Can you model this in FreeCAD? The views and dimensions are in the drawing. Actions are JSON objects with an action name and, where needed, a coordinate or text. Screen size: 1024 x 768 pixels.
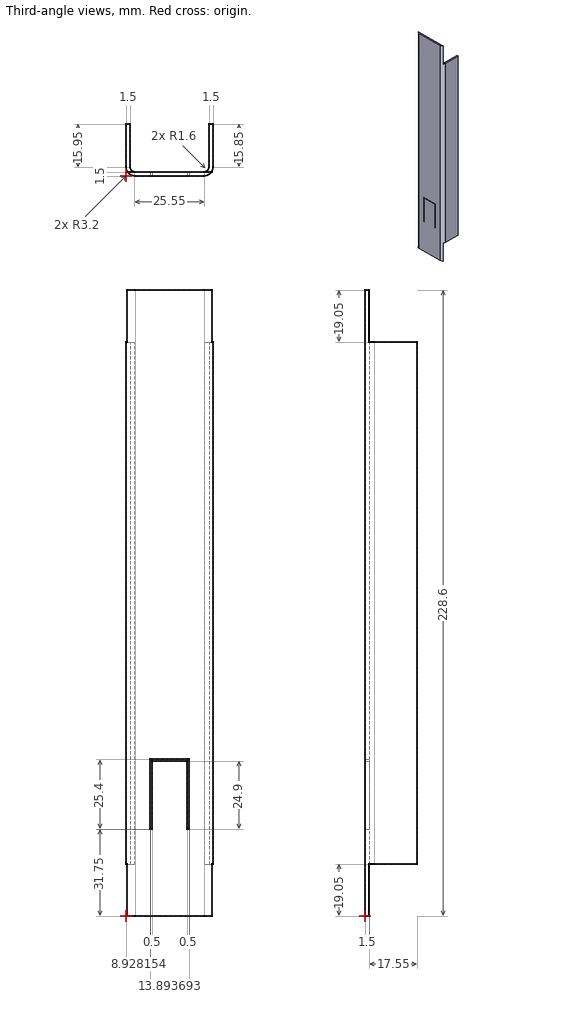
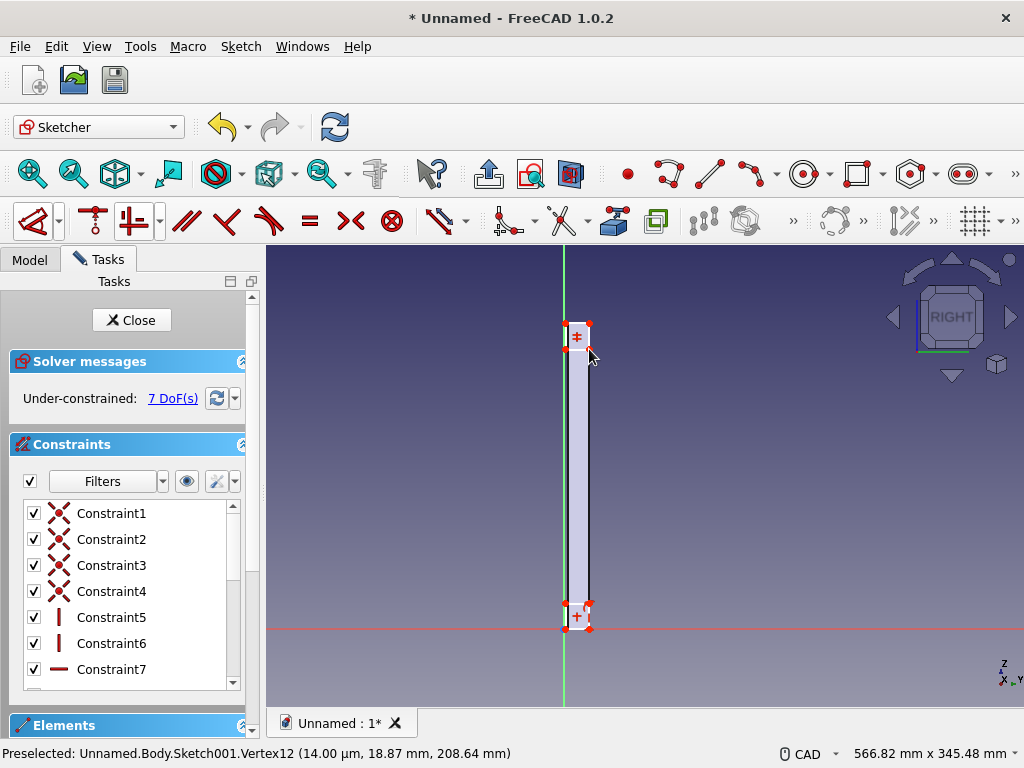
{"action": "scroll", "coordinate": [566, 604], "scroll_direction": "up", "scroll_amount": 15}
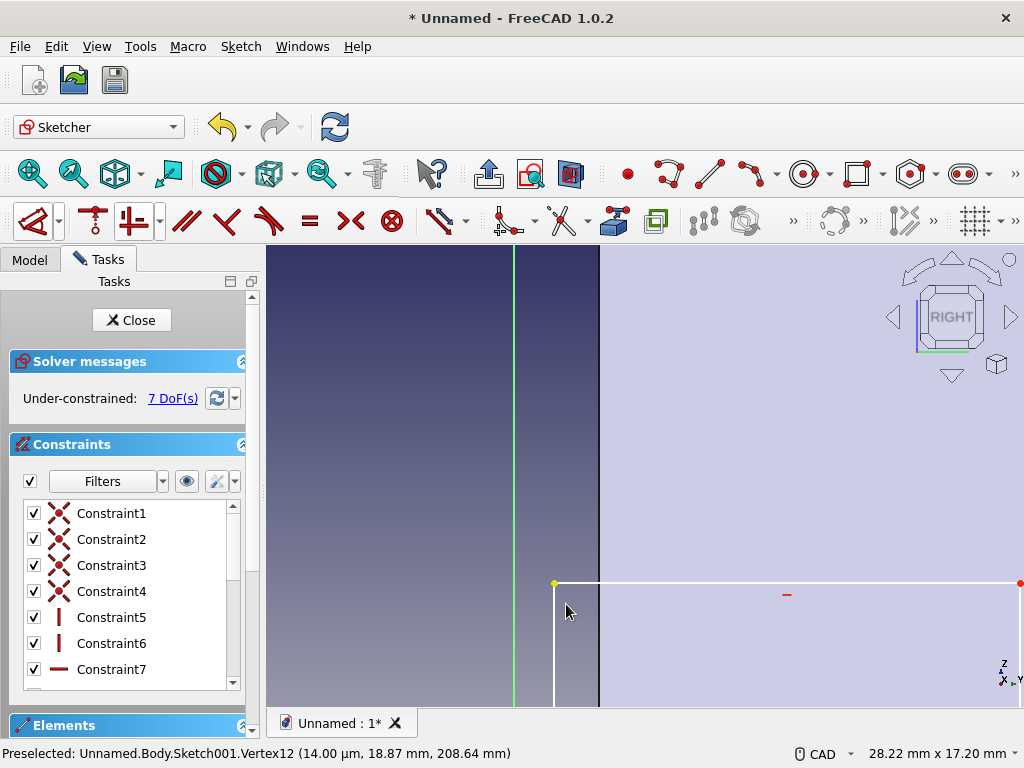
{"action": "left_click", "coordinate": [554, 583]}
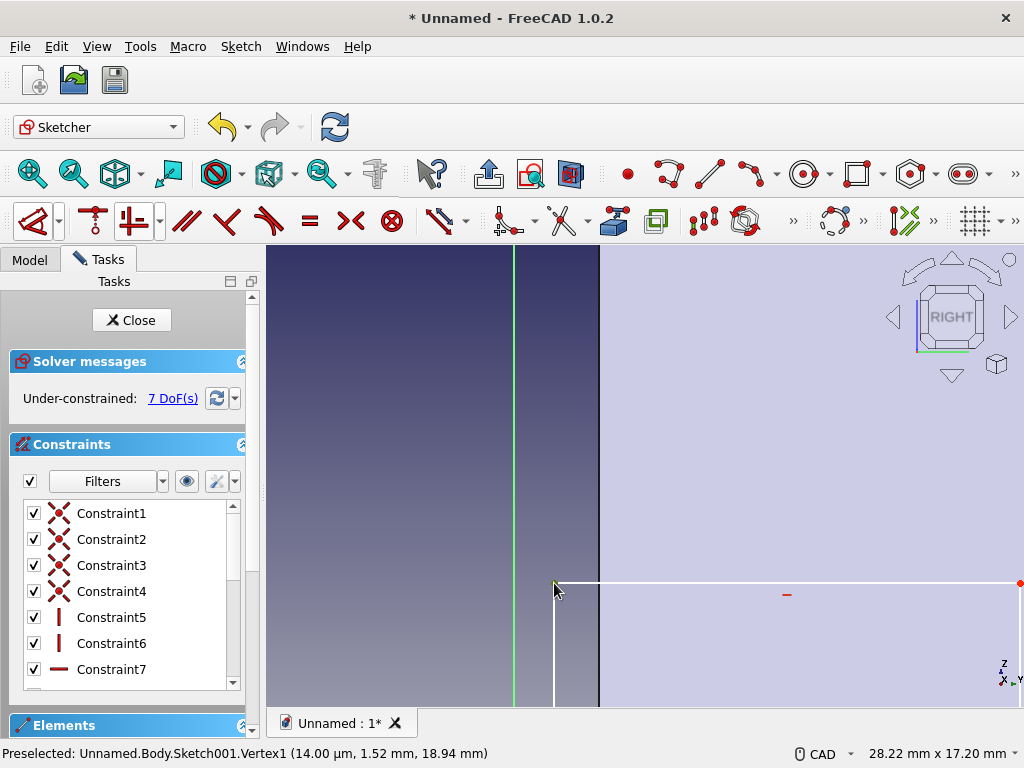
{"action": "key", "text": "l"}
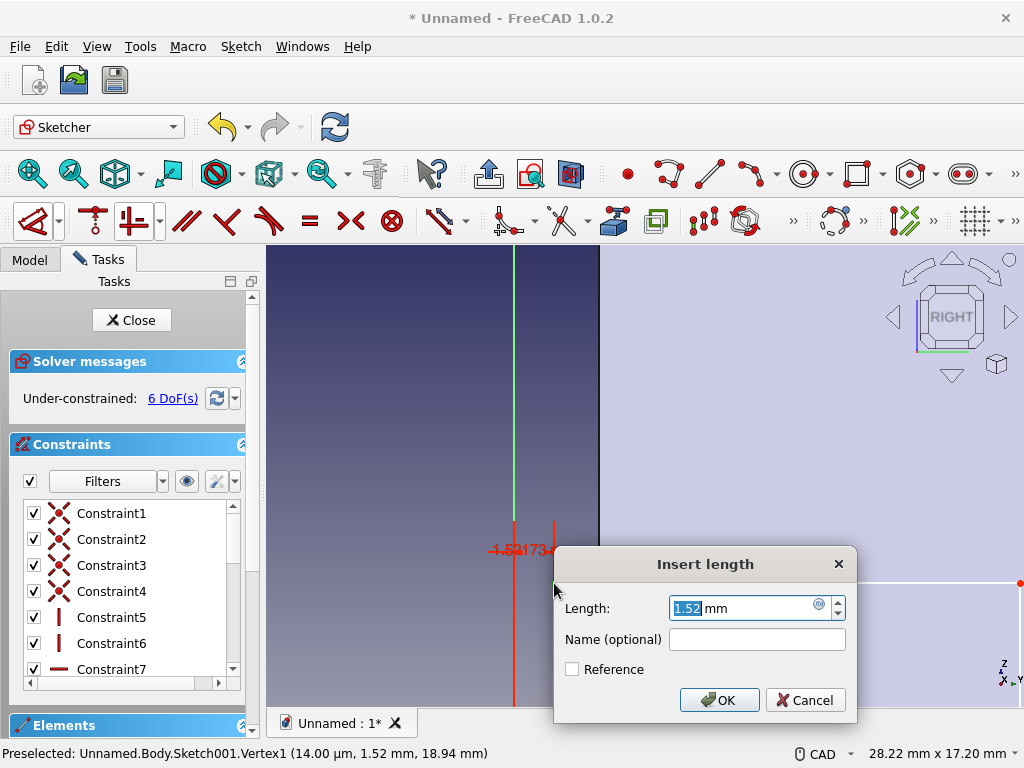
{"action": "type", "text": "1.5"}
{"action": "key", "text": "Return"}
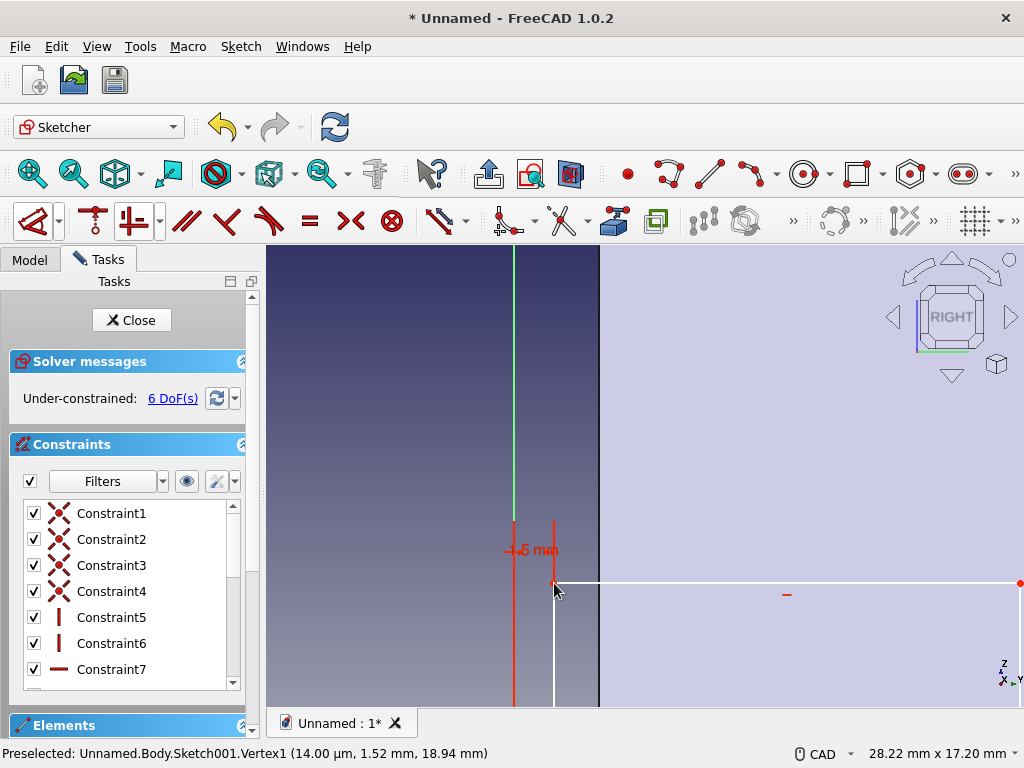
{"action": "scroll", "coordinate": [566, 605], "scroll_direction": "down", "scroll_amount": 15}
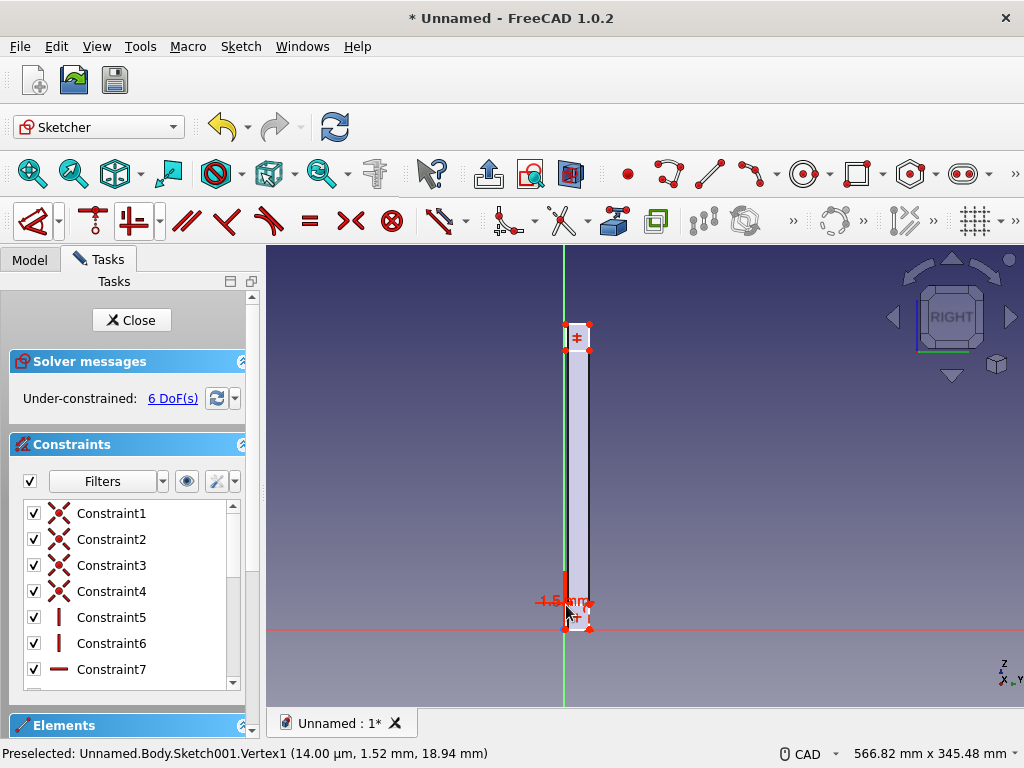
{"action": "scroll", "coordinate": [566, 324], "scroll_direction": "up", "scroll_amount": 15}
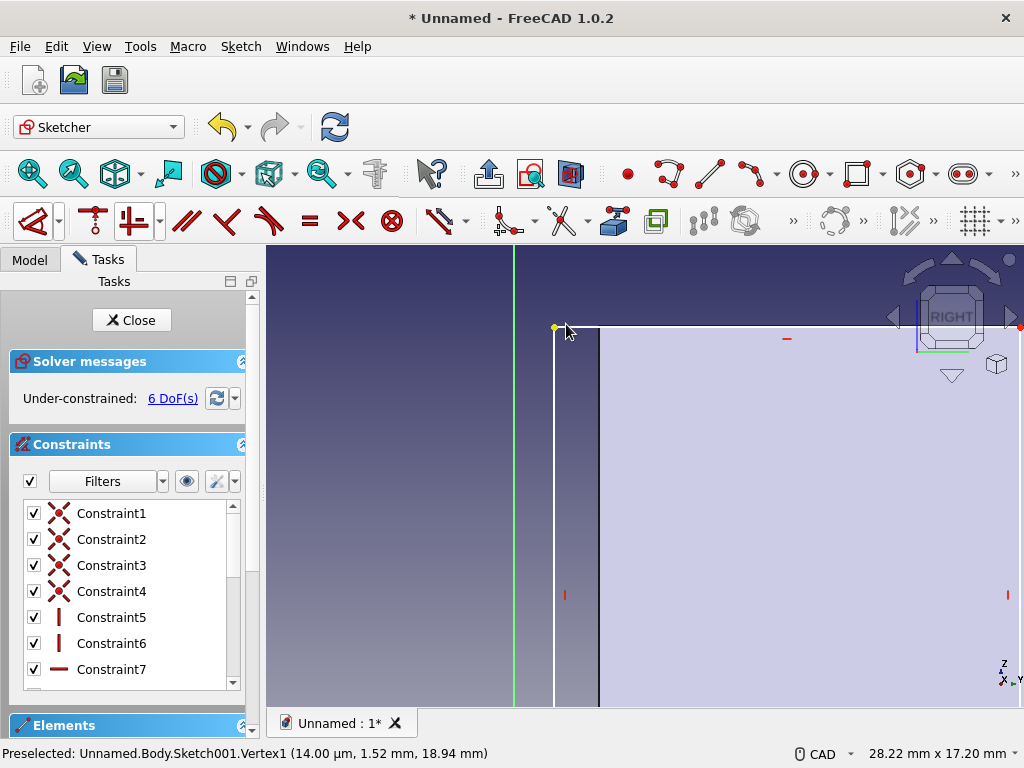
{"action": "left_click", "coordinate": [554, 327]}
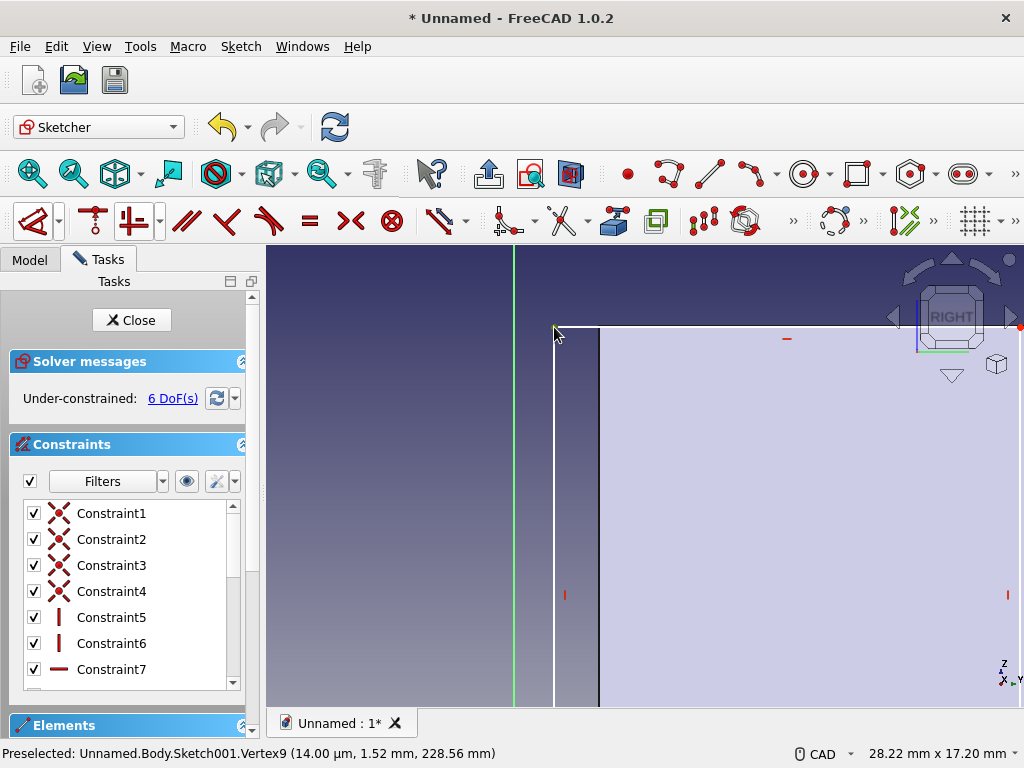
{"action": "key", "text": "l"}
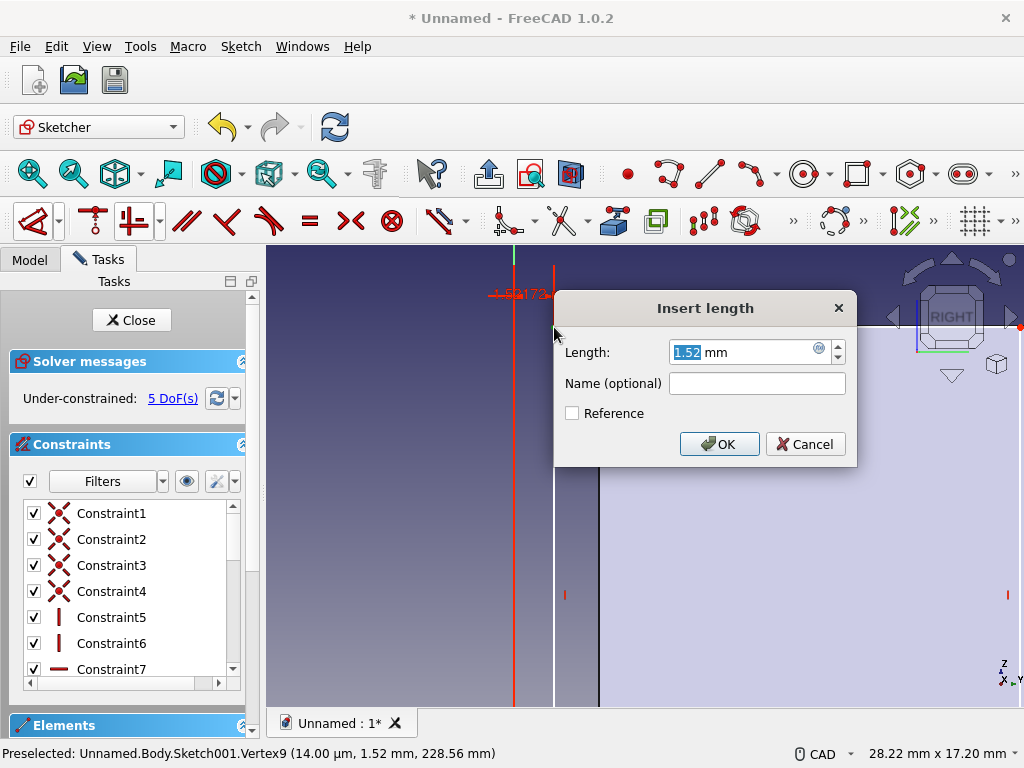
{"action": "type", "text": "1.5"}
{"action": "key", "text": "Return"}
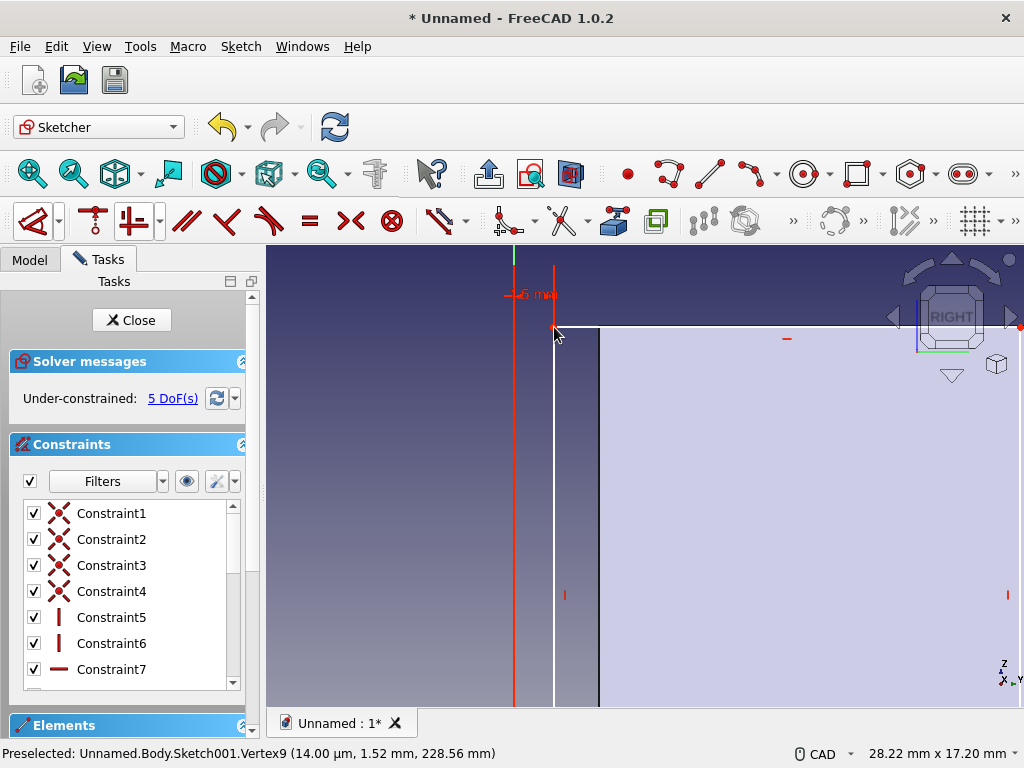
{"action": "scroll", "coordinate": [566, 323], "scroll_direction": "down", "scroll_amount": 15}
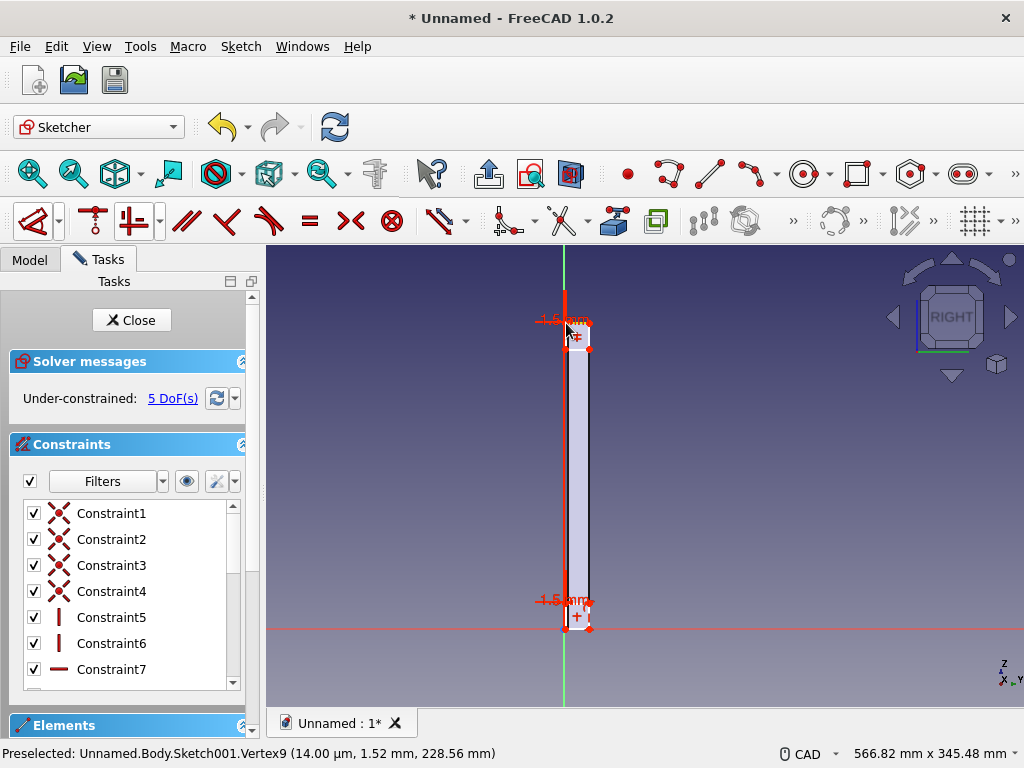
{"action": "scroll", "coordinate": [566, 611], "scroll_direction": "up", "scroll_amount": 10}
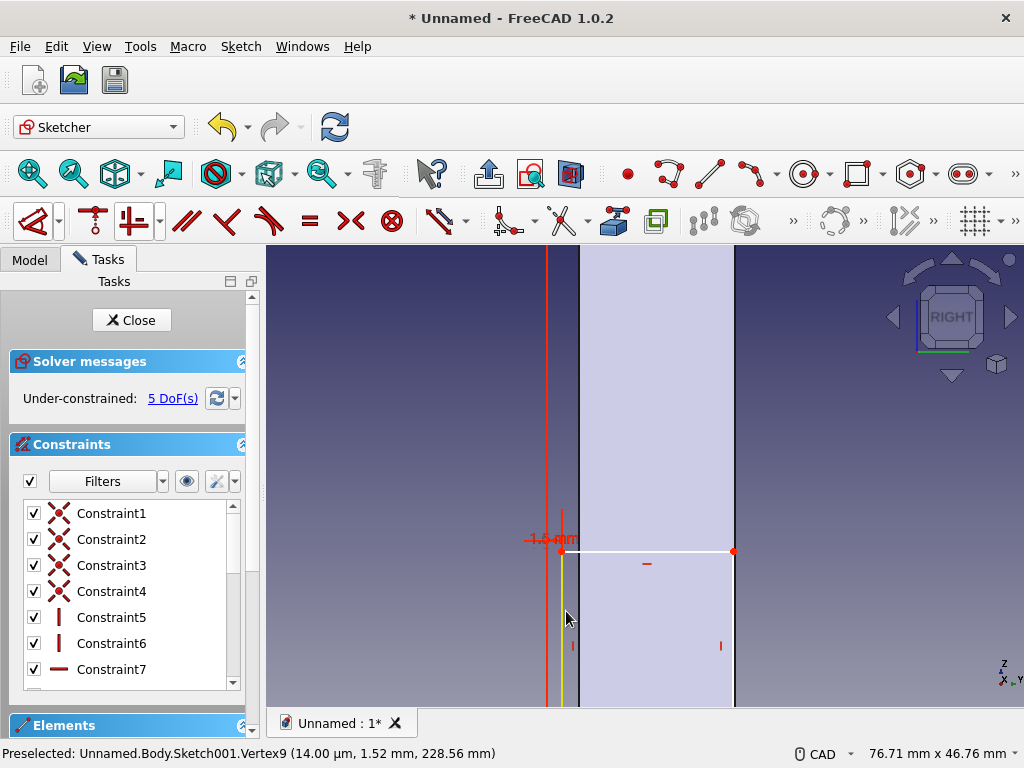
{"action": "left_click", "coordinate": [562, 608]}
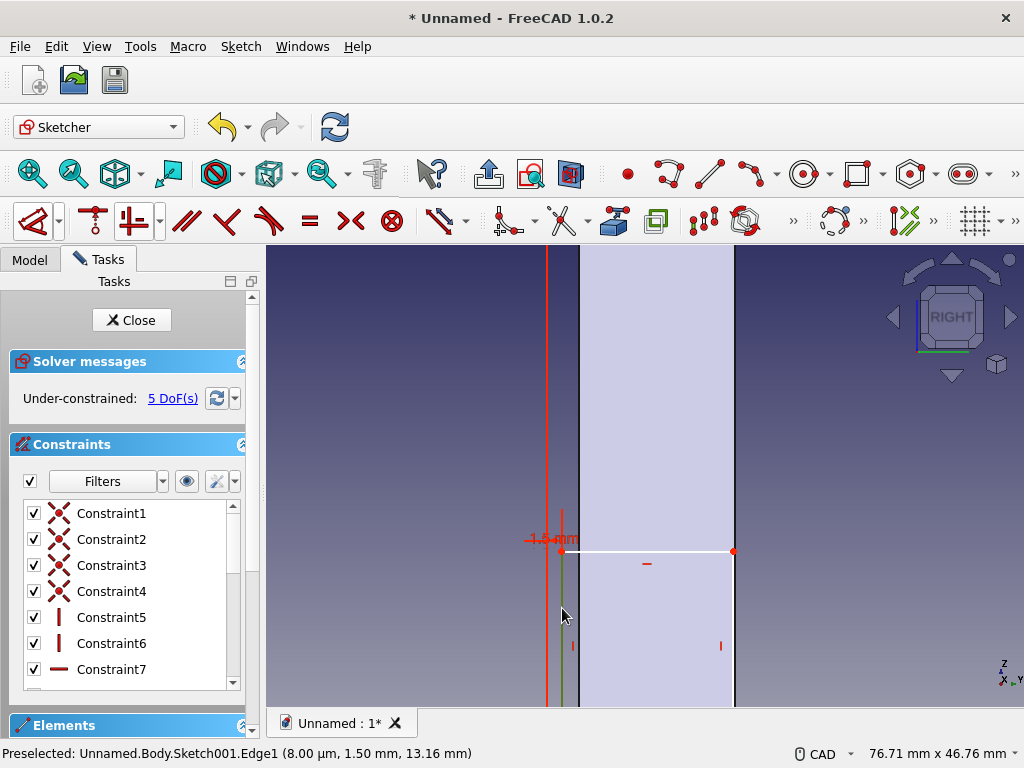
{"action": "key", "text": "i"}